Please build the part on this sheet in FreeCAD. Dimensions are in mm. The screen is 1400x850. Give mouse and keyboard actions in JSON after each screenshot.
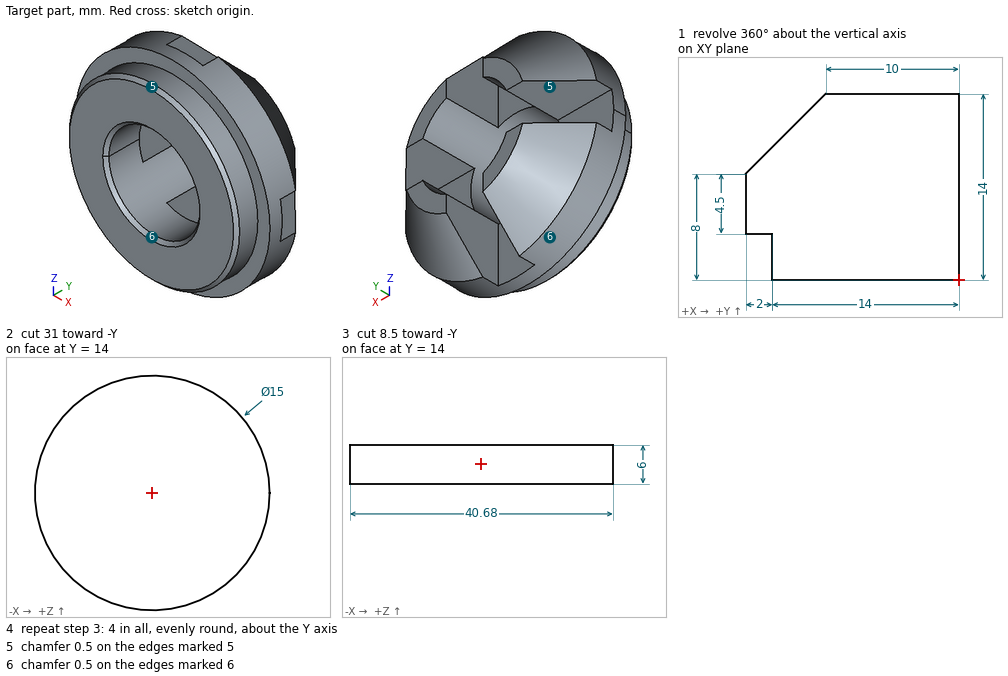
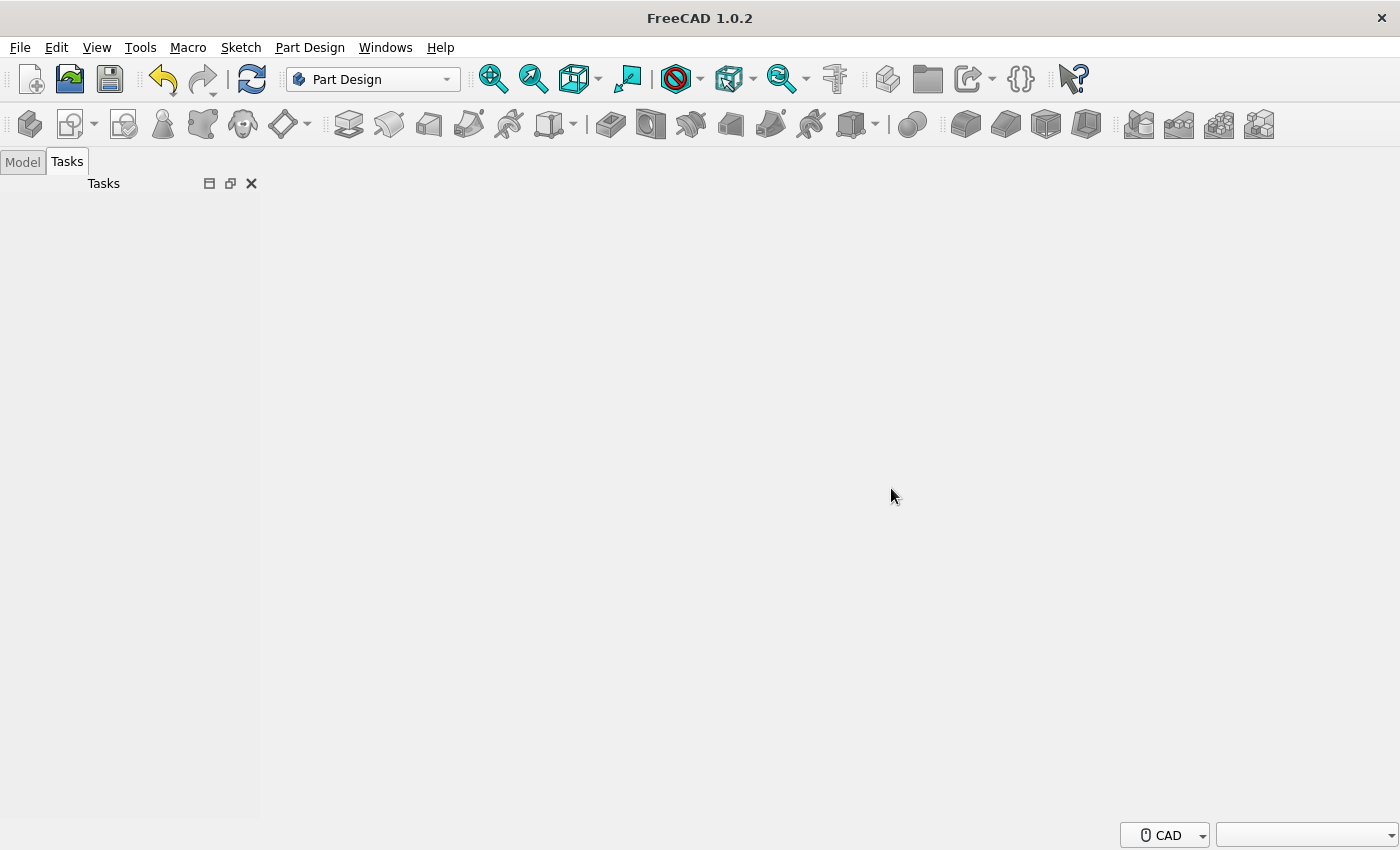
{"action": "left_click", "coordinate": [30, 80]}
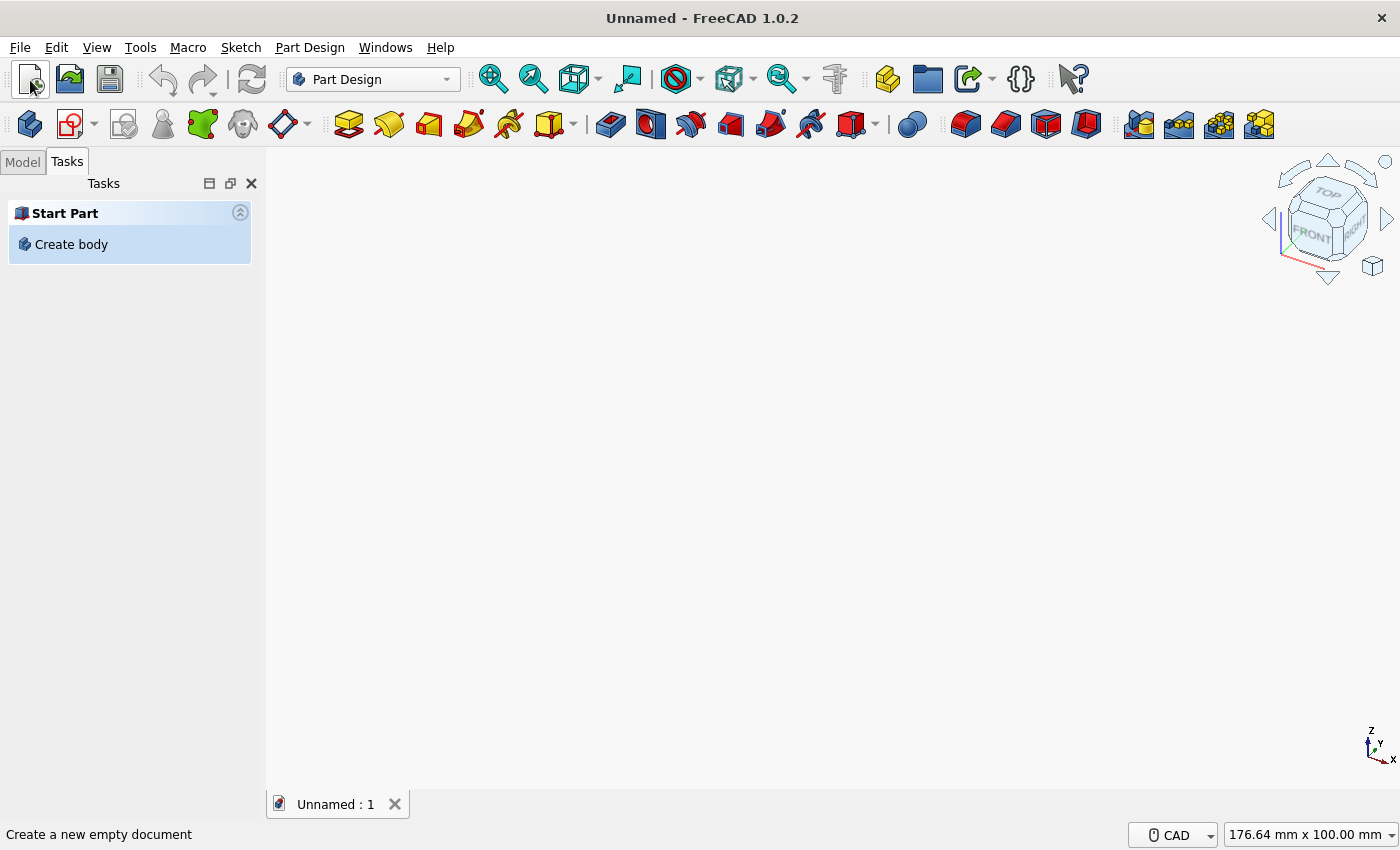
{"action": "left_click", "coordinate": [70, 124]}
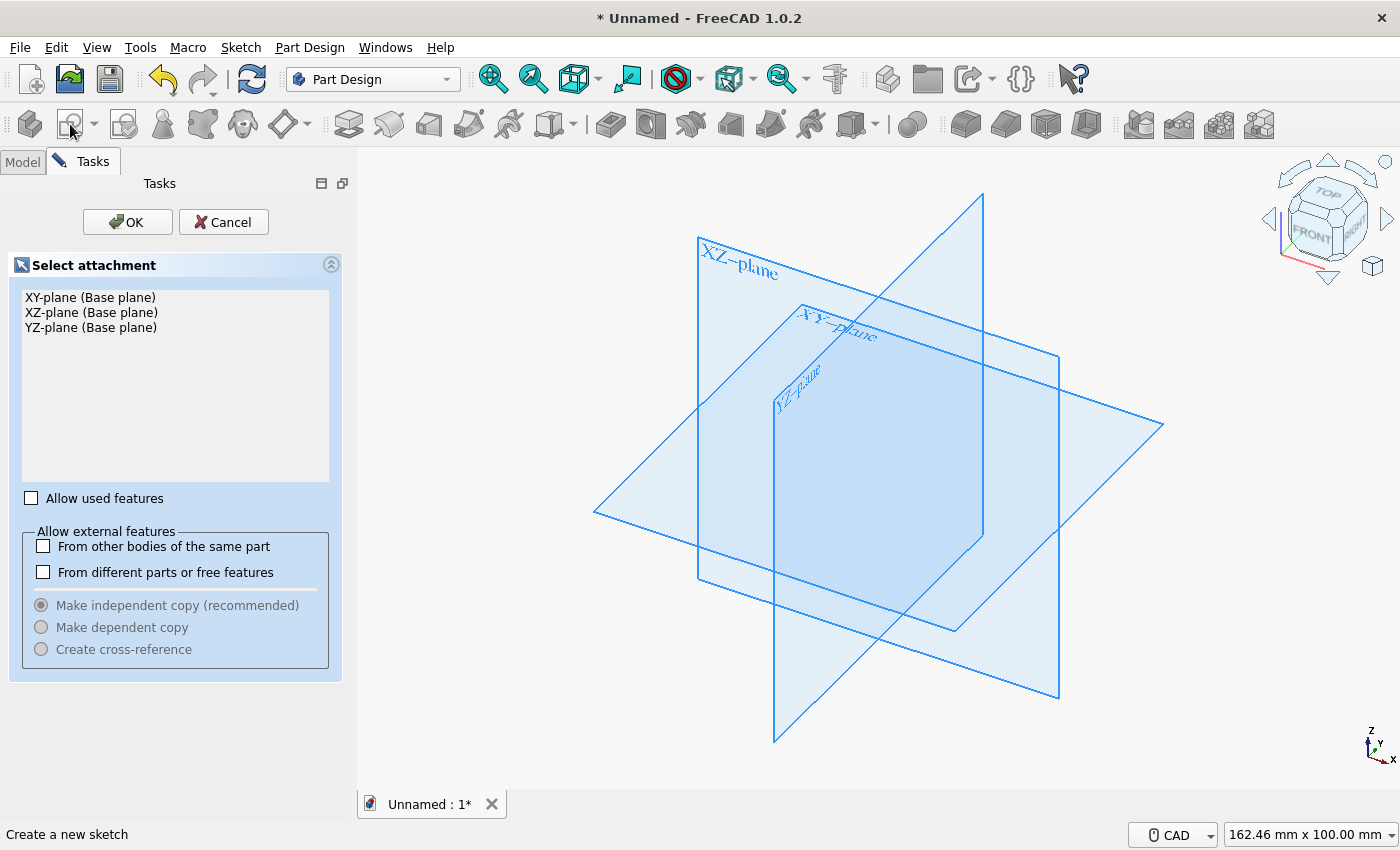
{"action": "left_click", "coordinate": [82, 298]}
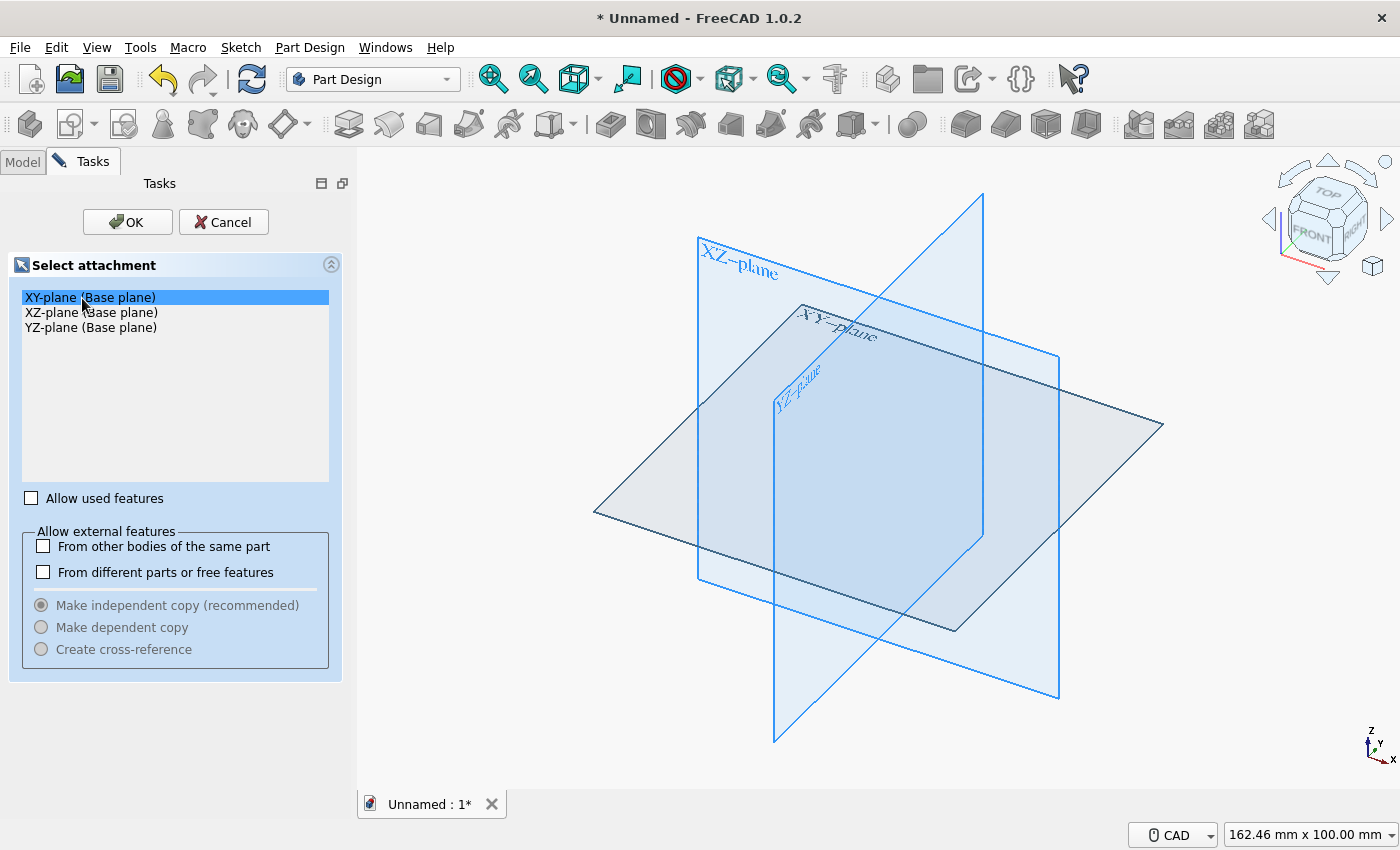
{"action": "left_click", "coordinate": [128, 222]}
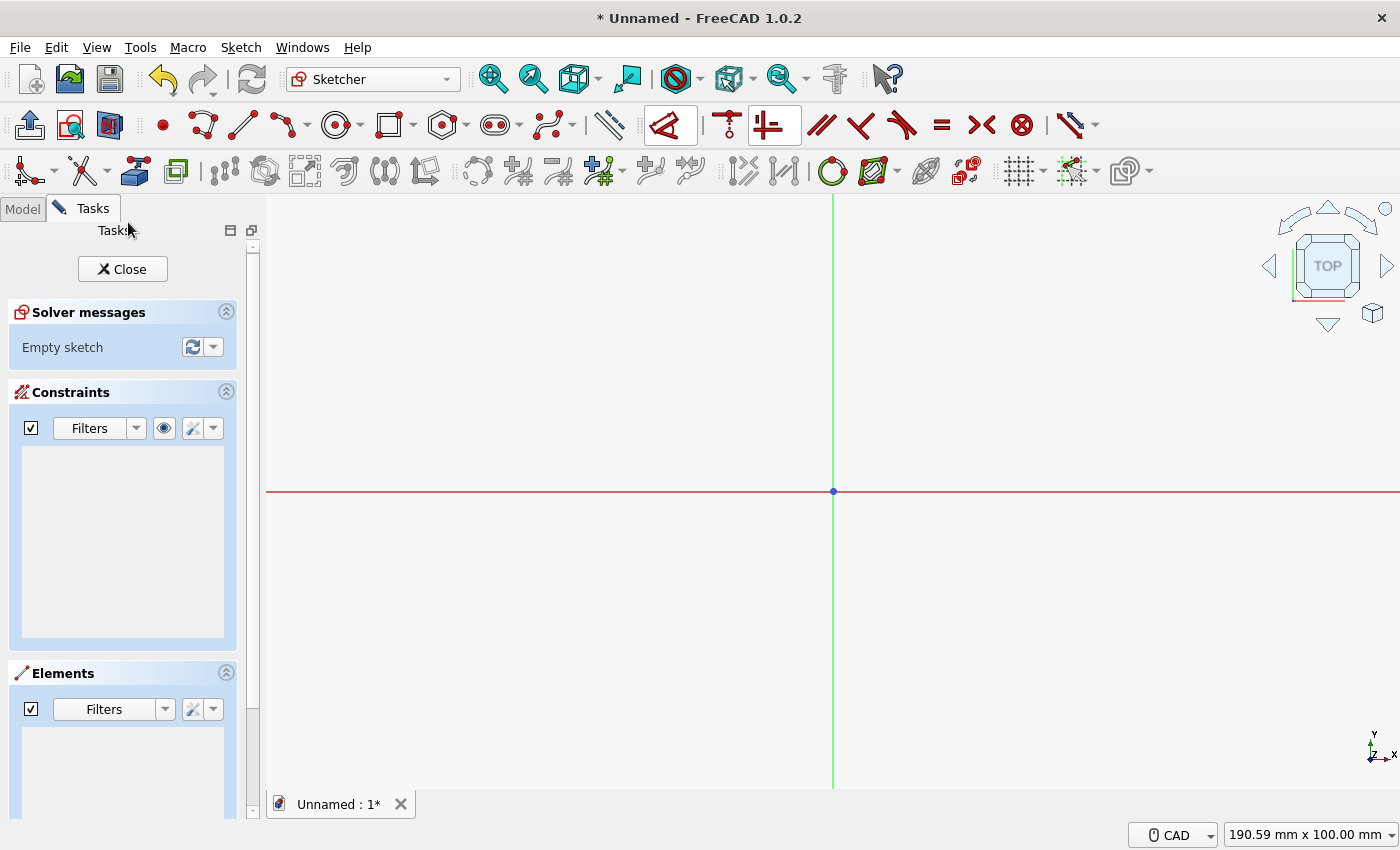
{"action": "scroll", "coordinate": [791, 439], "scroll_direction": "up", "scroll_amount": 8}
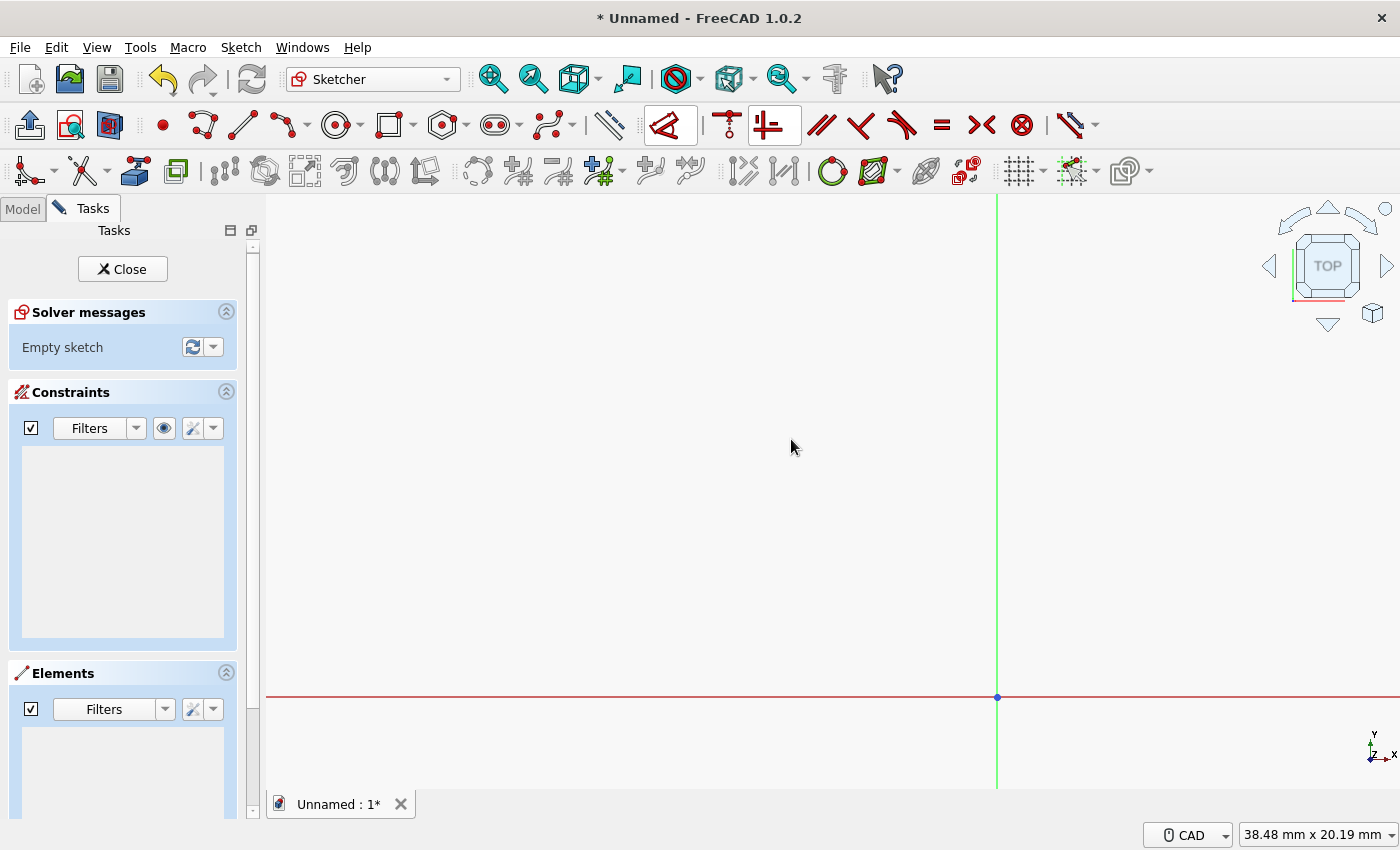
{"action": "left_click", "coordinate": [204, 126]}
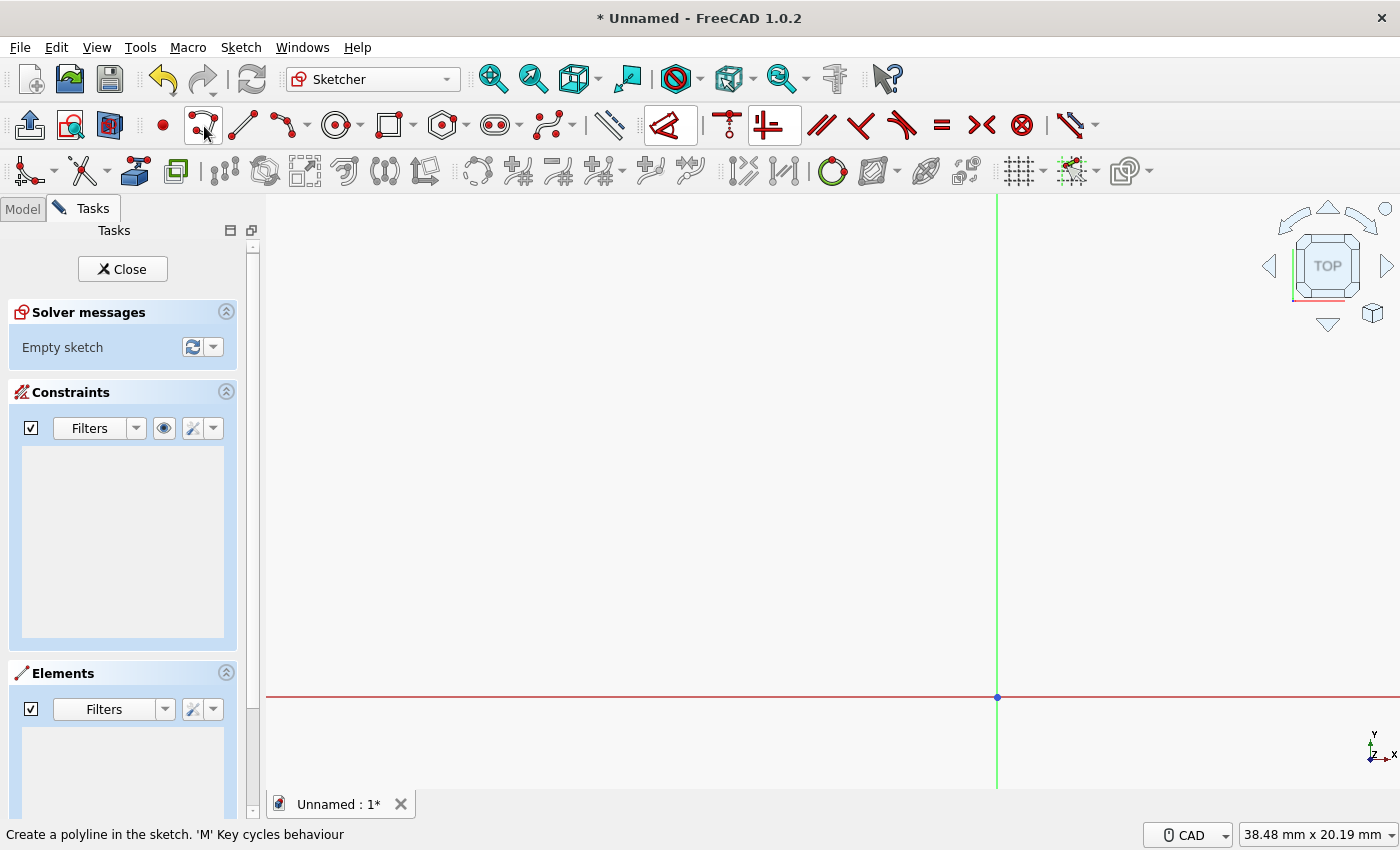
{"action": "left_click", "coordinate": [997, 697]}
{"action": "left_click", "coordinate": [988, 285]}
{"action": "left_click", "coordinate": [702, 285]}
{"action": "left_click", "coordinate": [526, 462]}
{"action": "left_click", "coordinate": [526, 594]}
{"action": "left_click", "coordinate": [585, 594]}
{"action": "left_click", "coordinate": [585, 688]}
{"action": "left_click", "coordinate": [997, 697]}
{"action": "key", "text": "Escape"}
{"action": "key", "text": "Escape"}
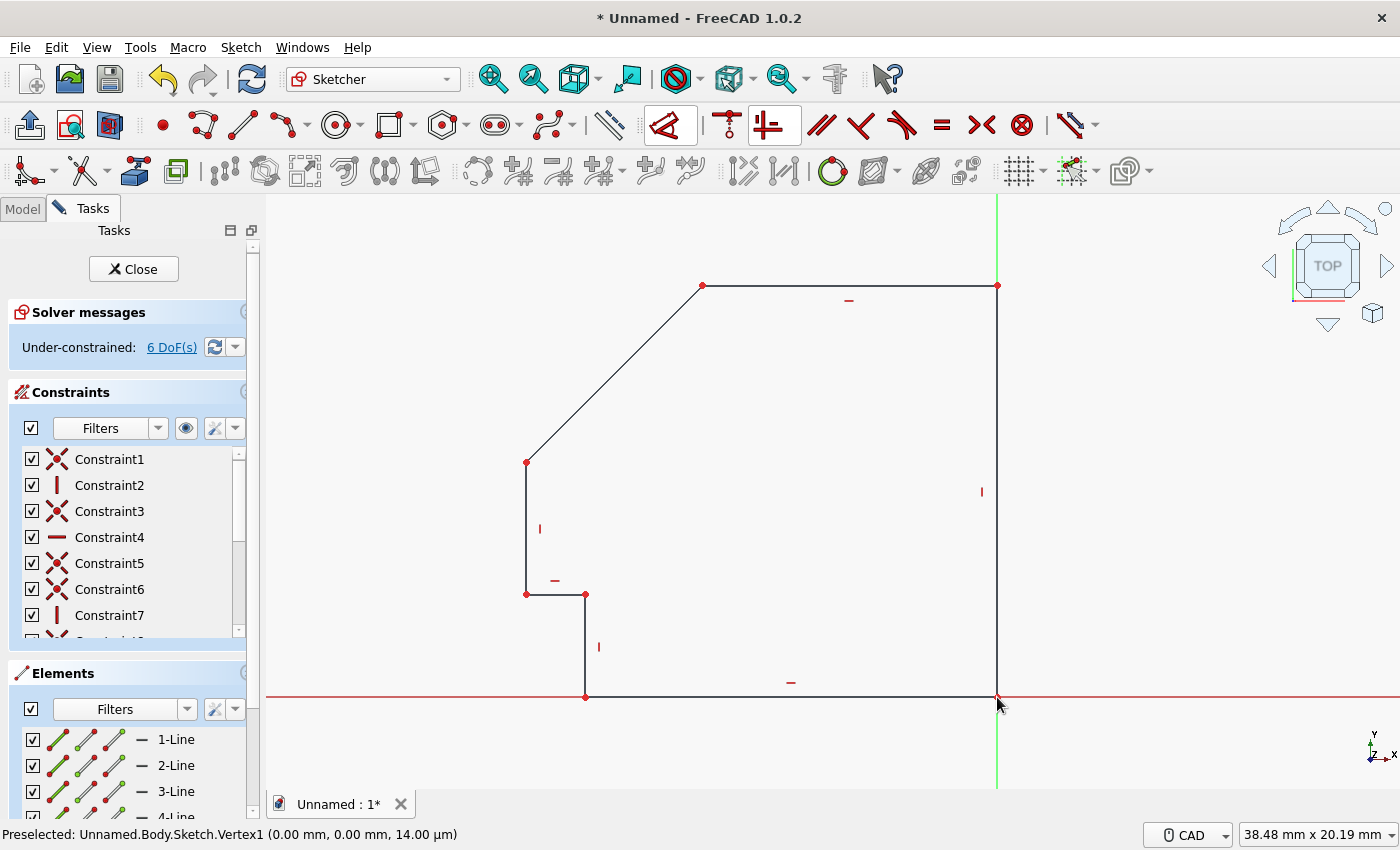
{"action": "left_click", "coordinate": [664, 126]}